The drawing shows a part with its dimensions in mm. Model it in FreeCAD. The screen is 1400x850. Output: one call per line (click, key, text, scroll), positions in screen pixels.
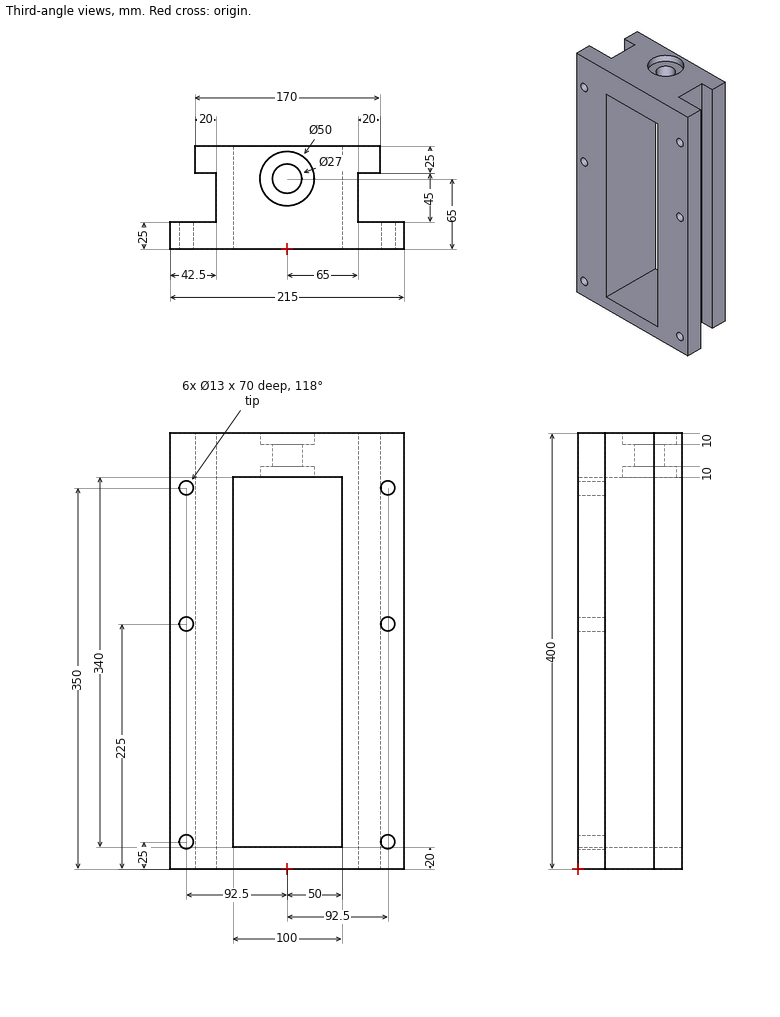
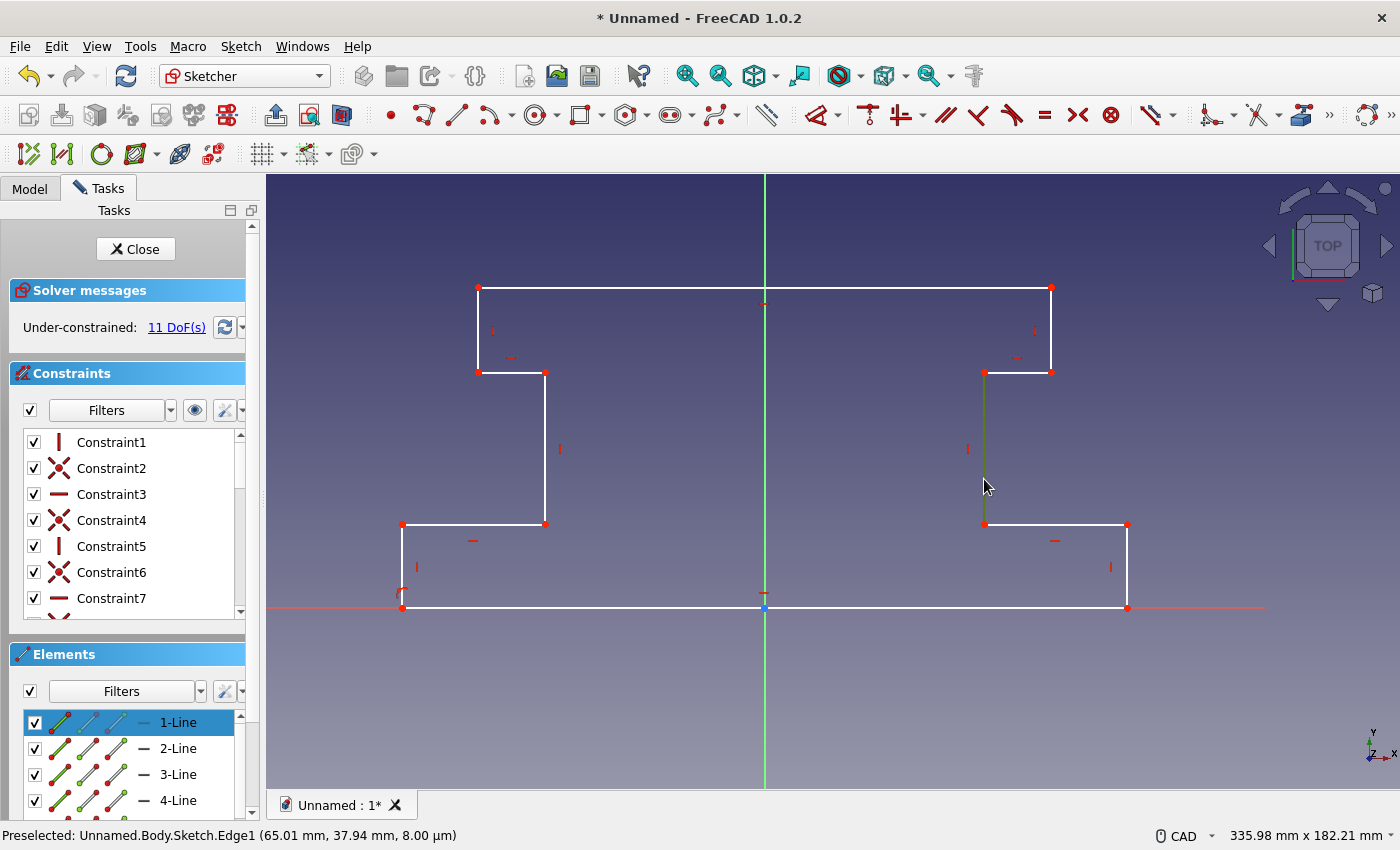
click(838, 116)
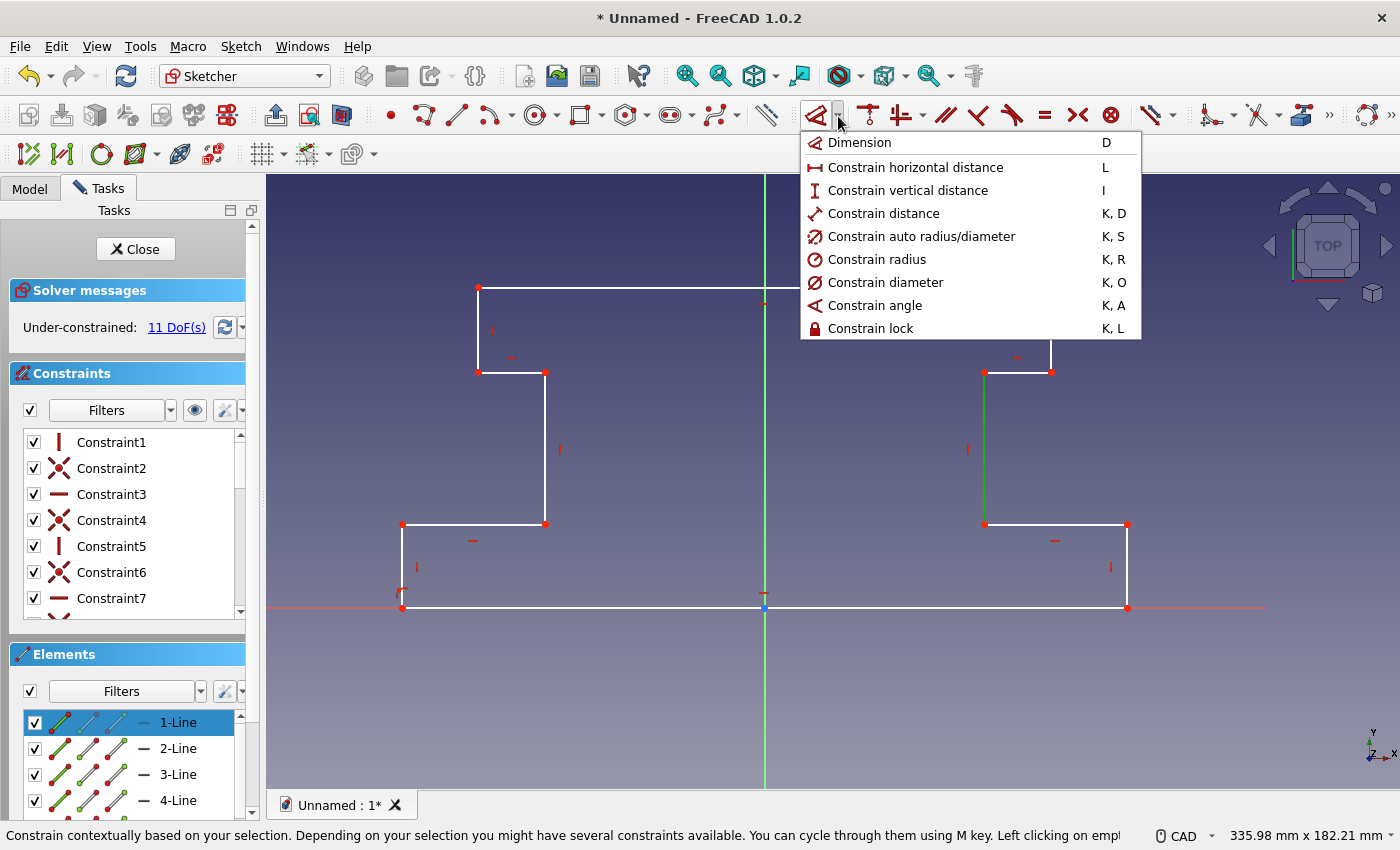
click(971, 190)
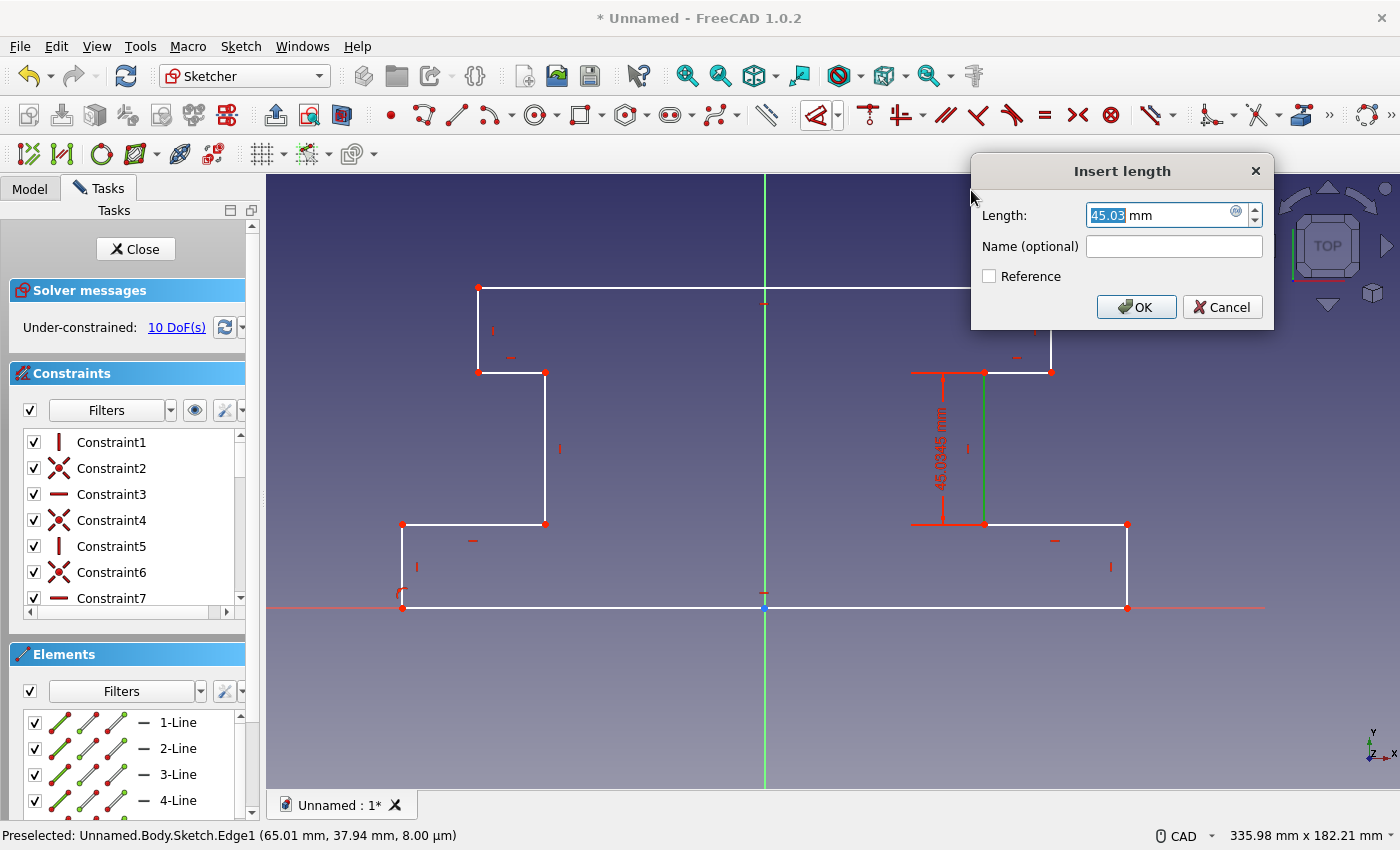
text(45)
key(Return)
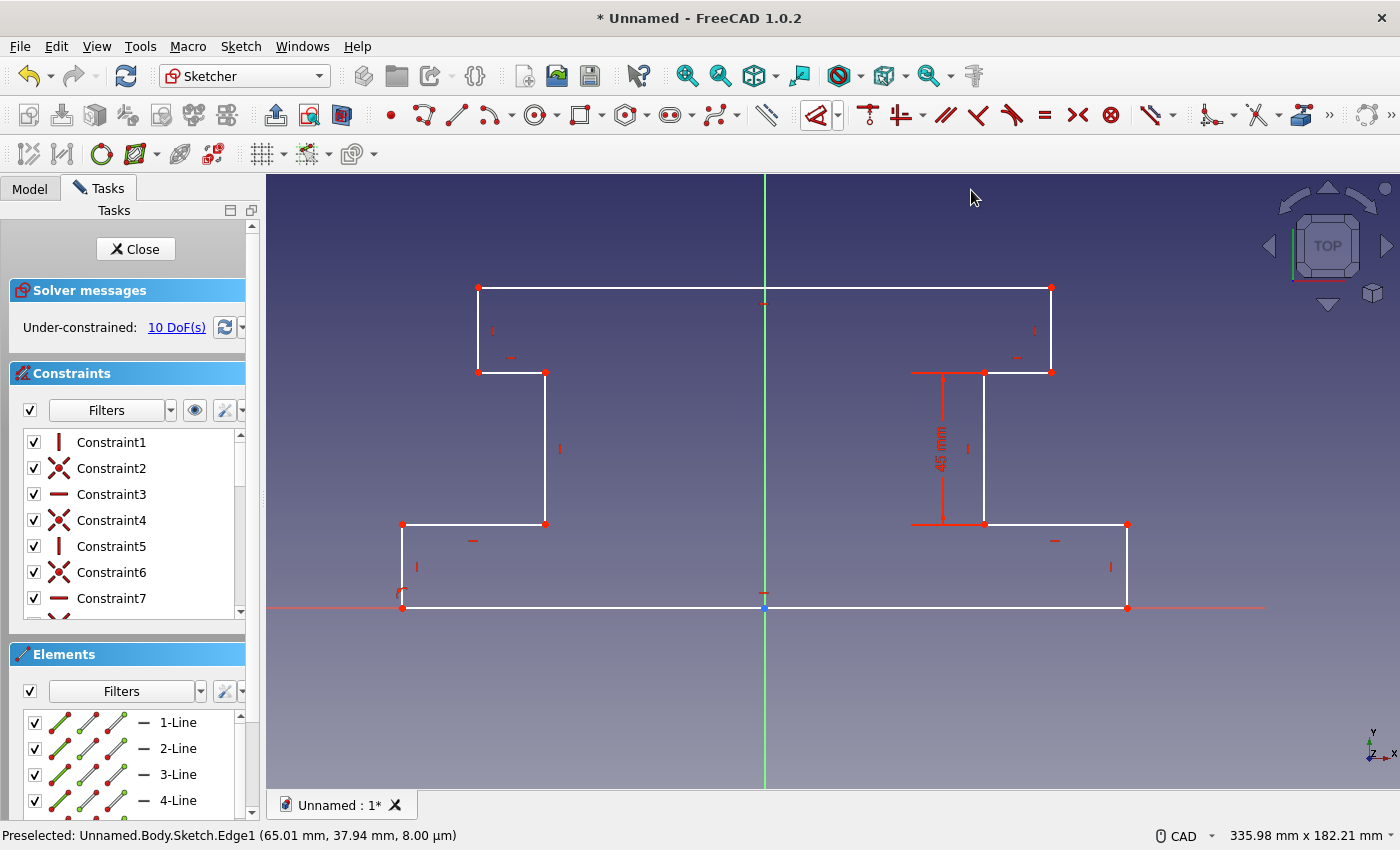
click(1004, 373)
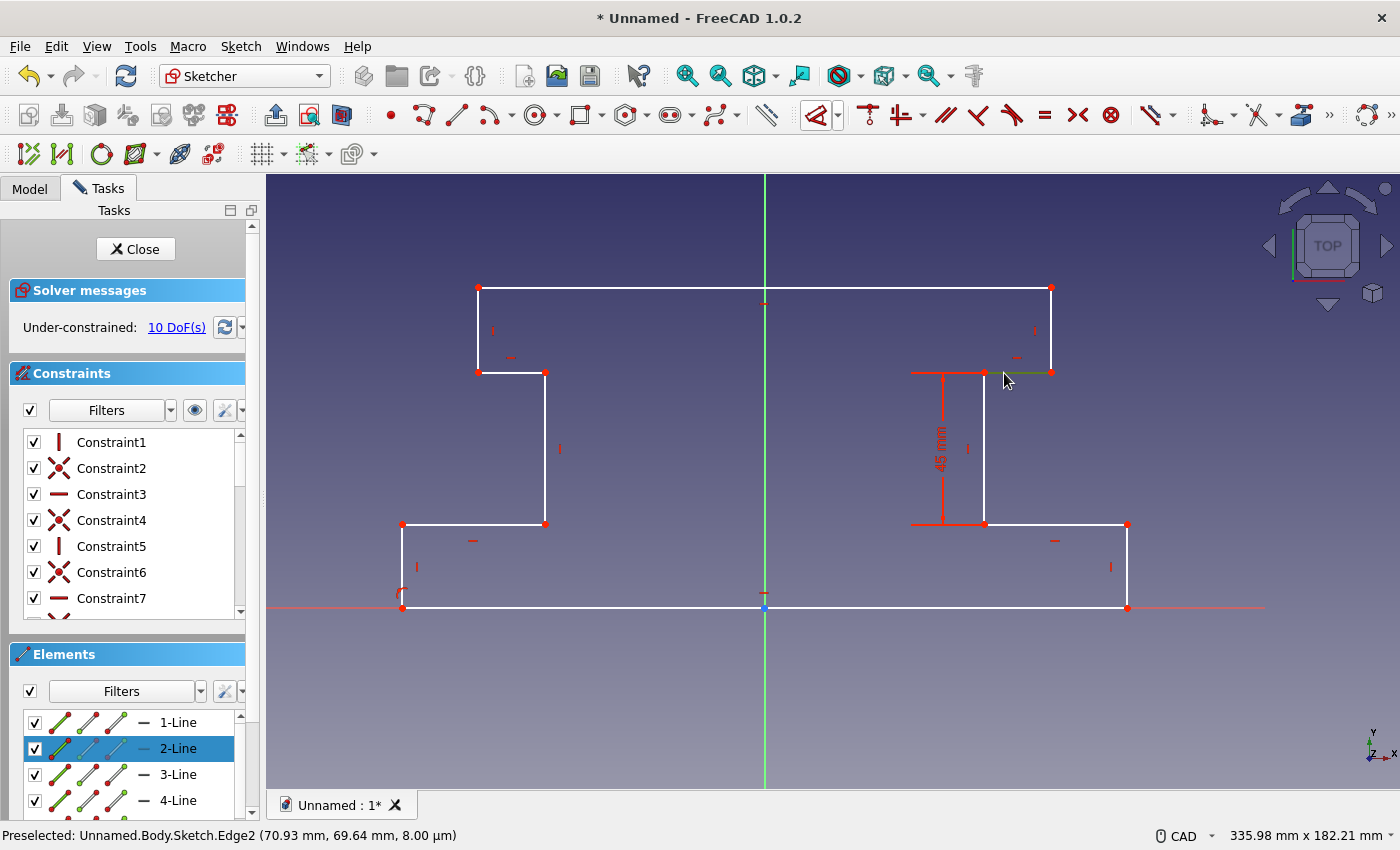
key(l)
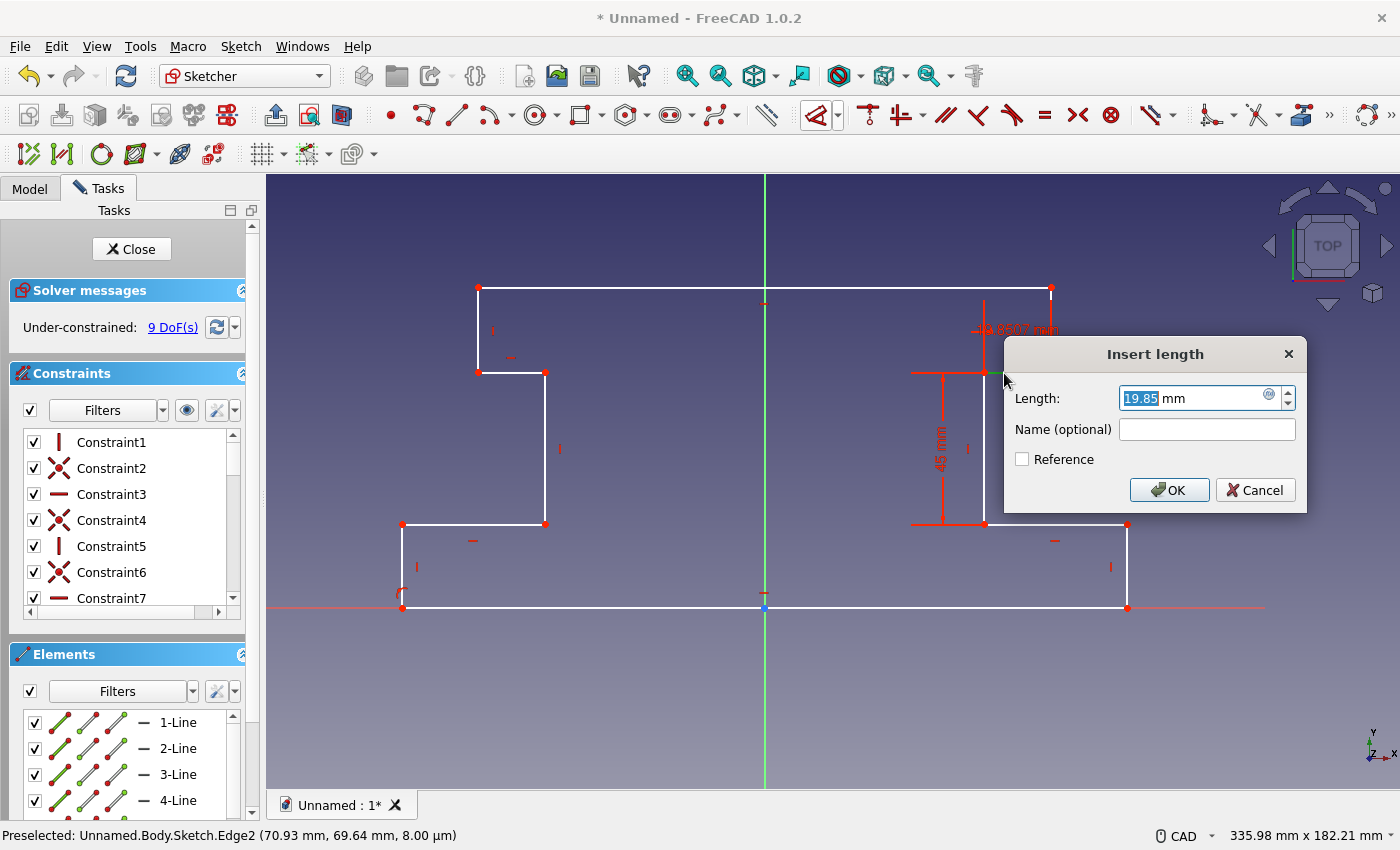
text(20)
key(Return)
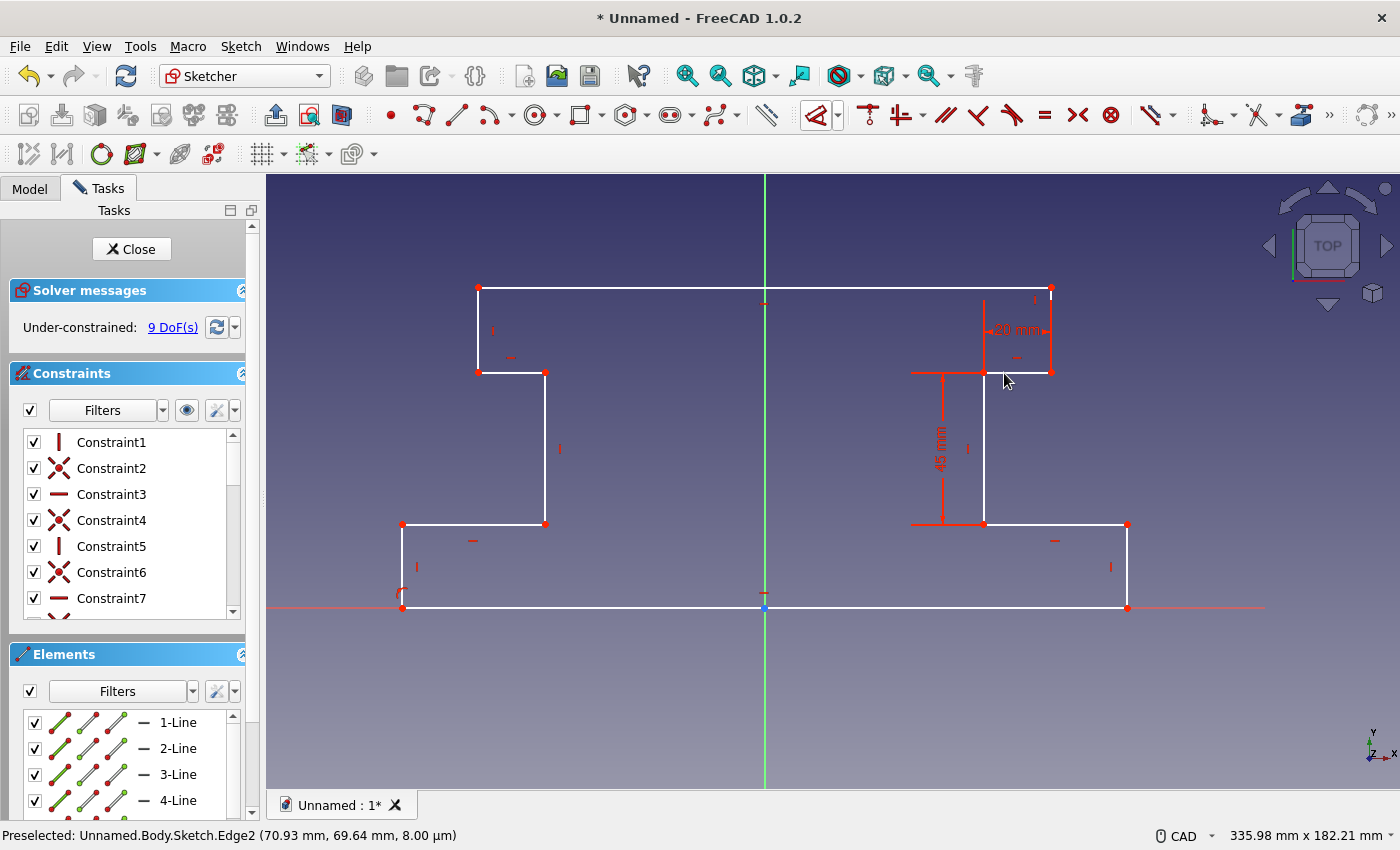
click(1051, 348)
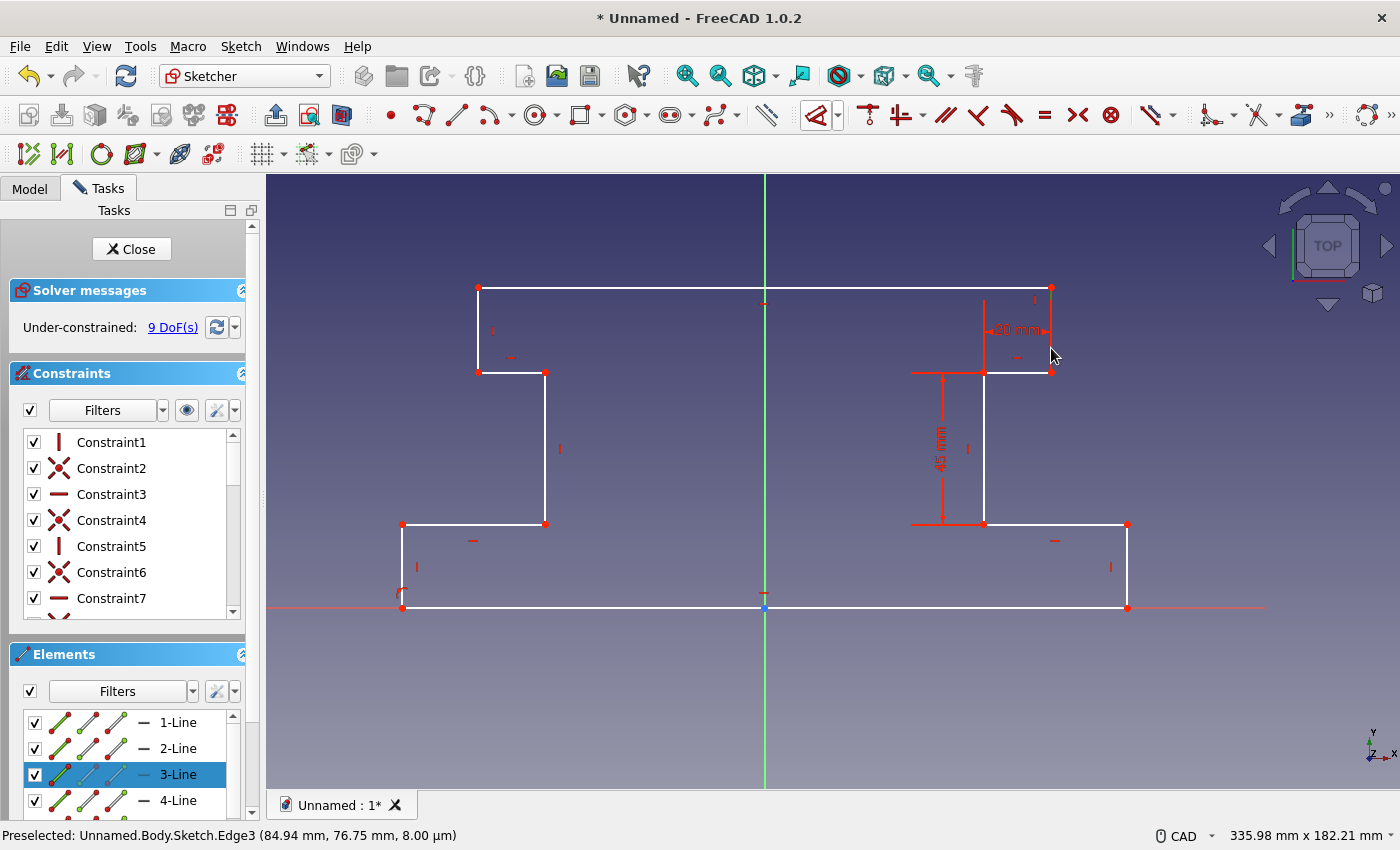
key(i)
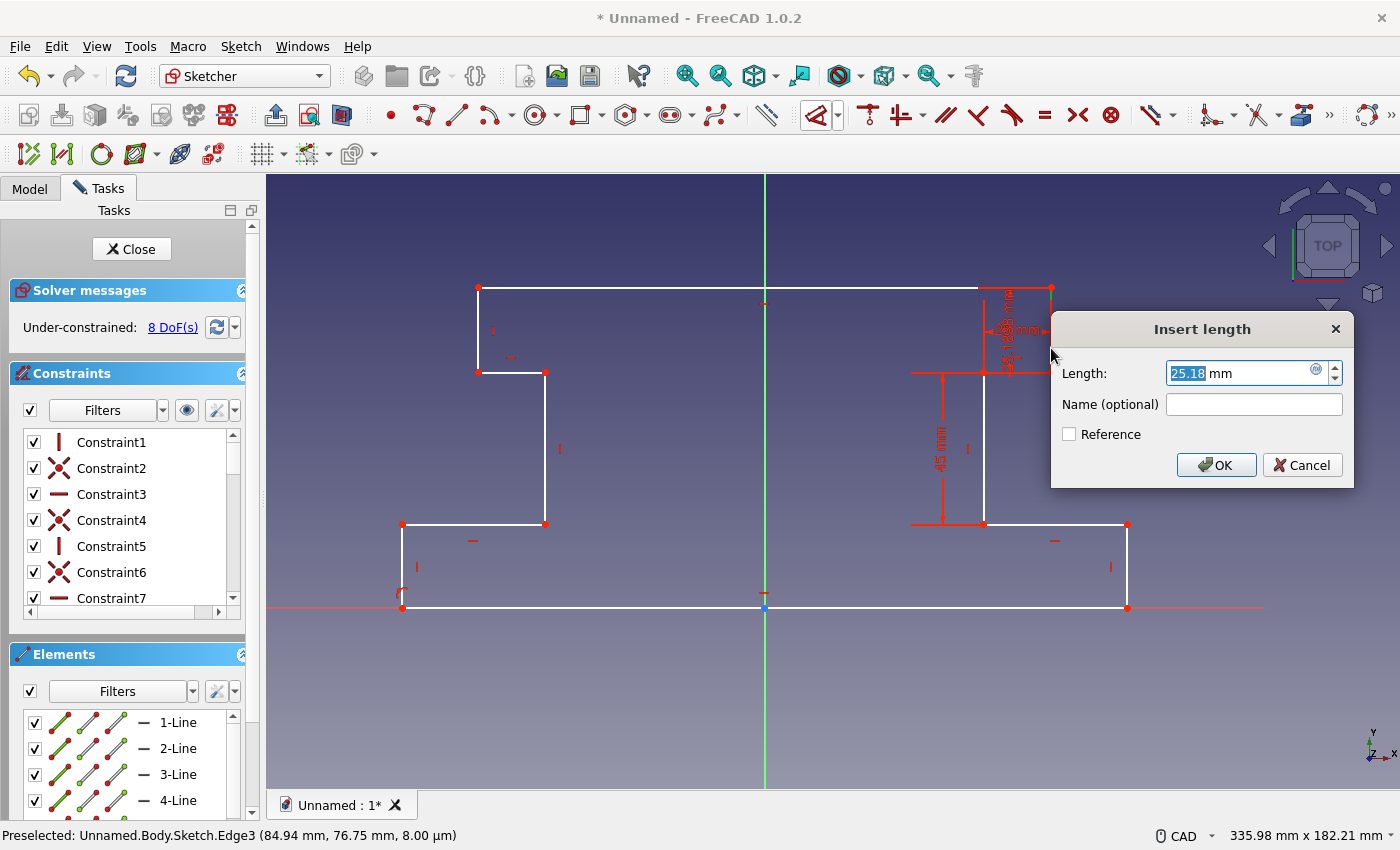
text(25)
key(Return)